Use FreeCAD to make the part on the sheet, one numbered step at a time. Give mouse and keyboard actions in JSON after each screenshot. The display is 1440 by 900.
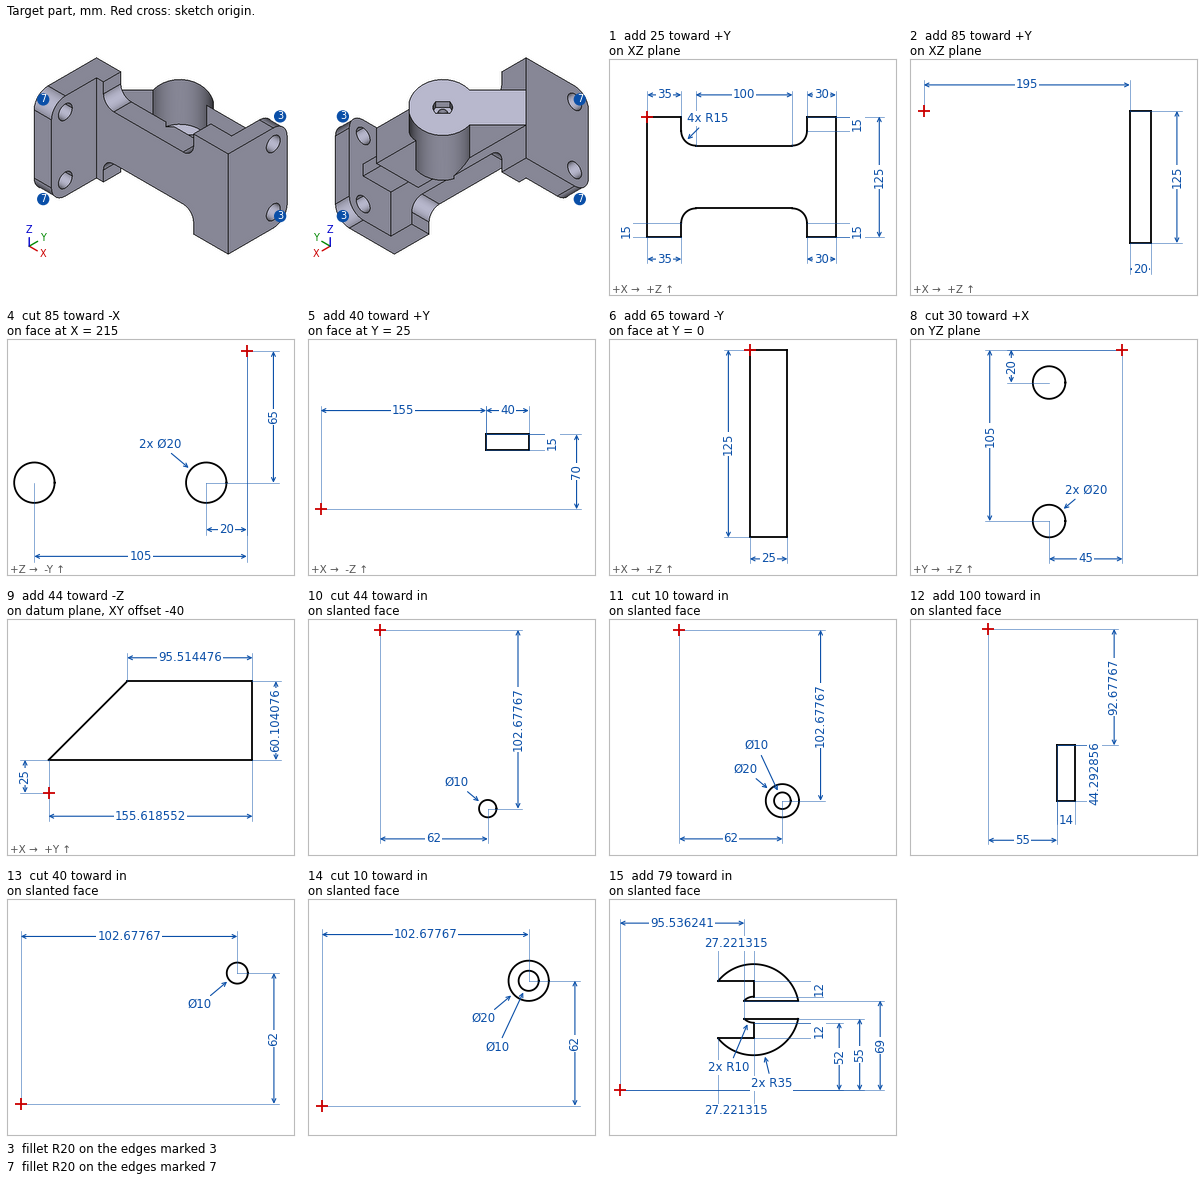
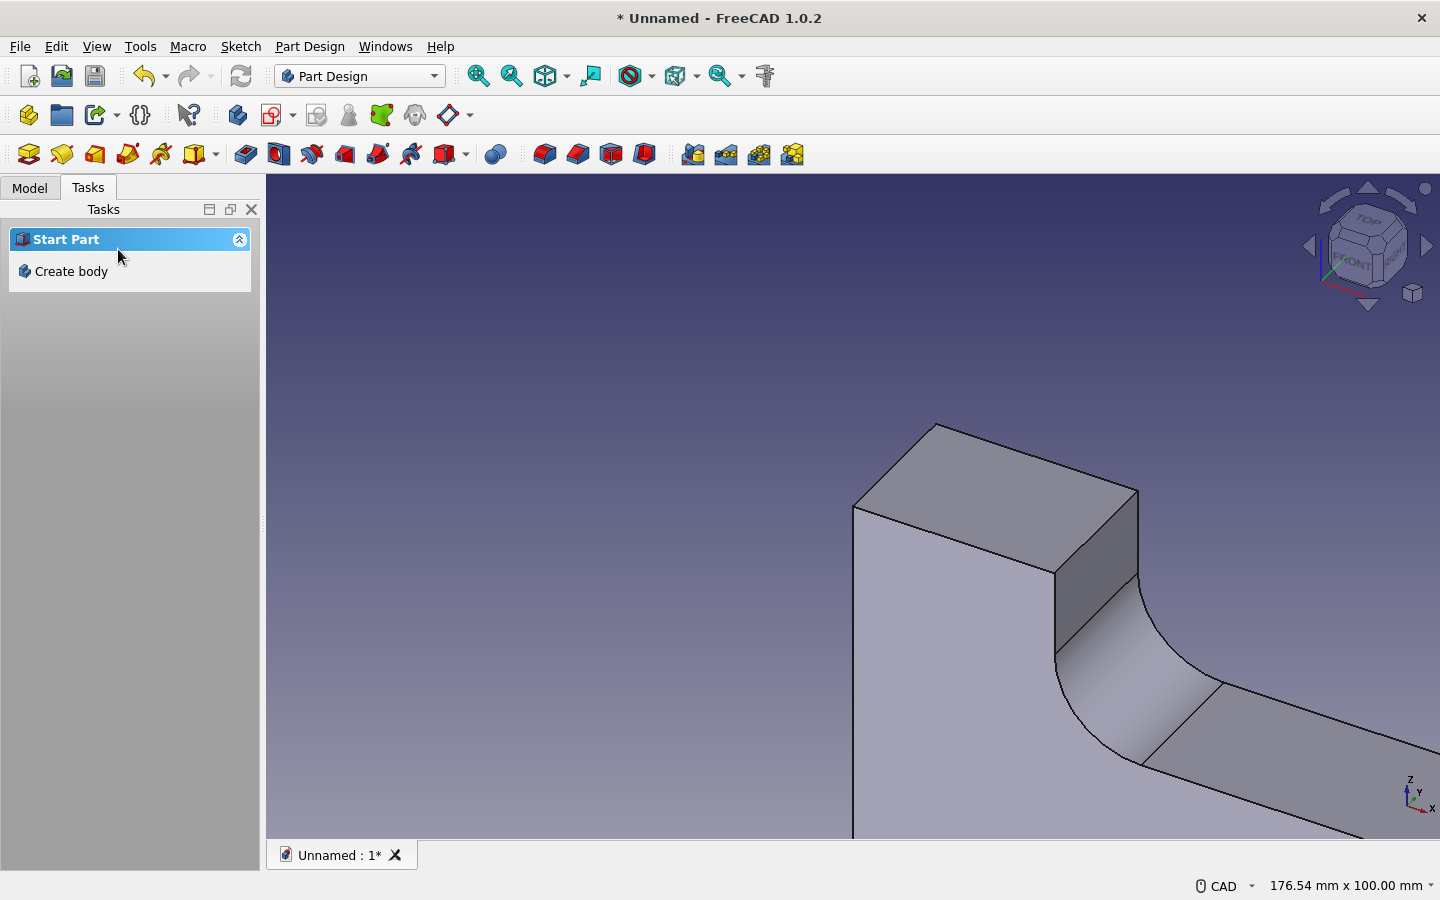
{"action": "left_click", "coordinate": [479, 76]}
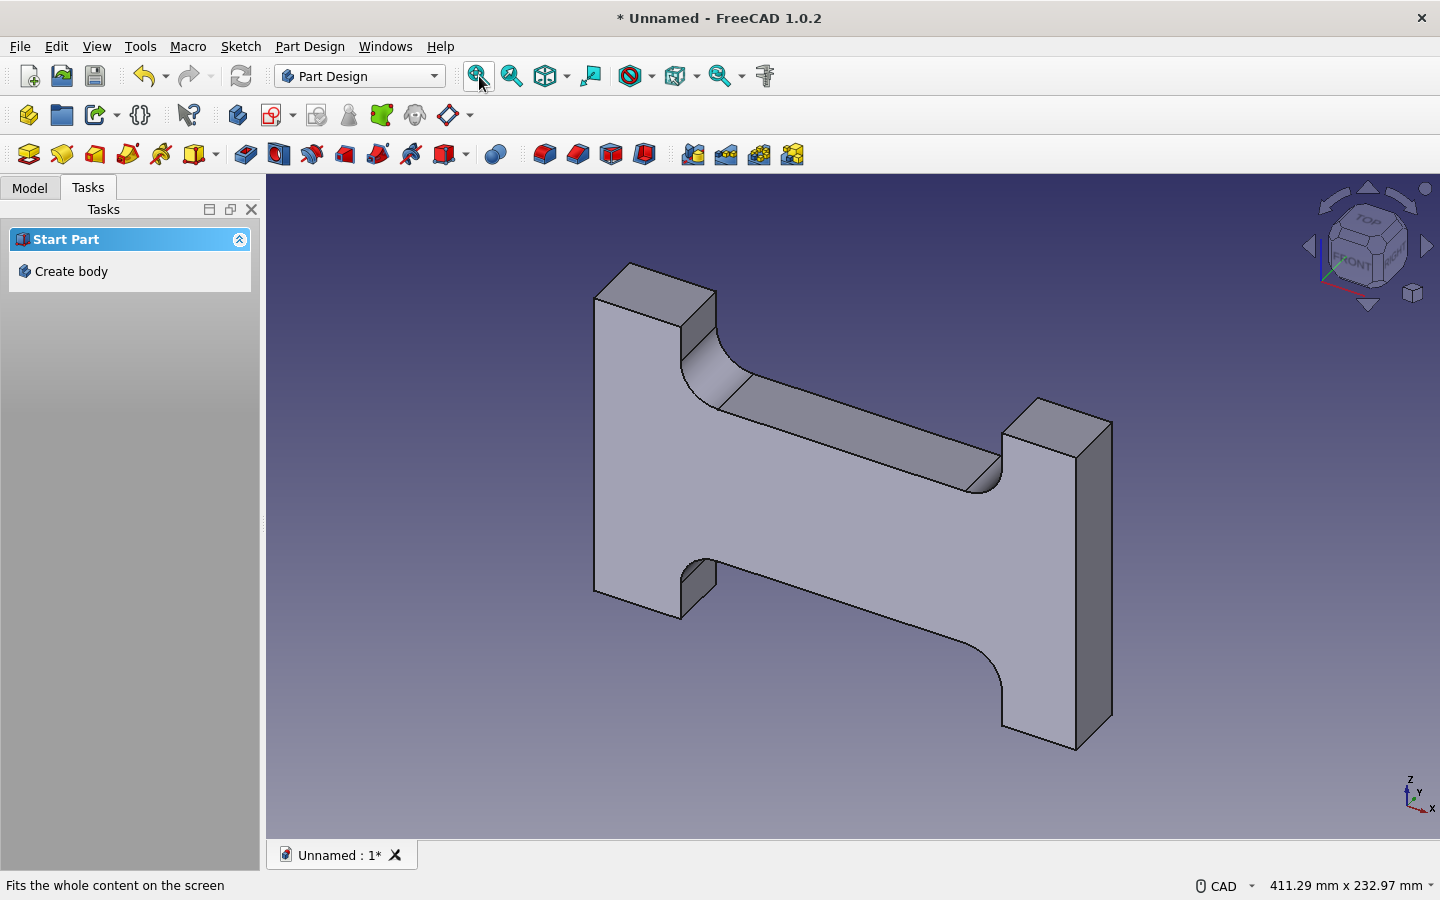
{"action": "left_click", "coordinate": [270, 116]}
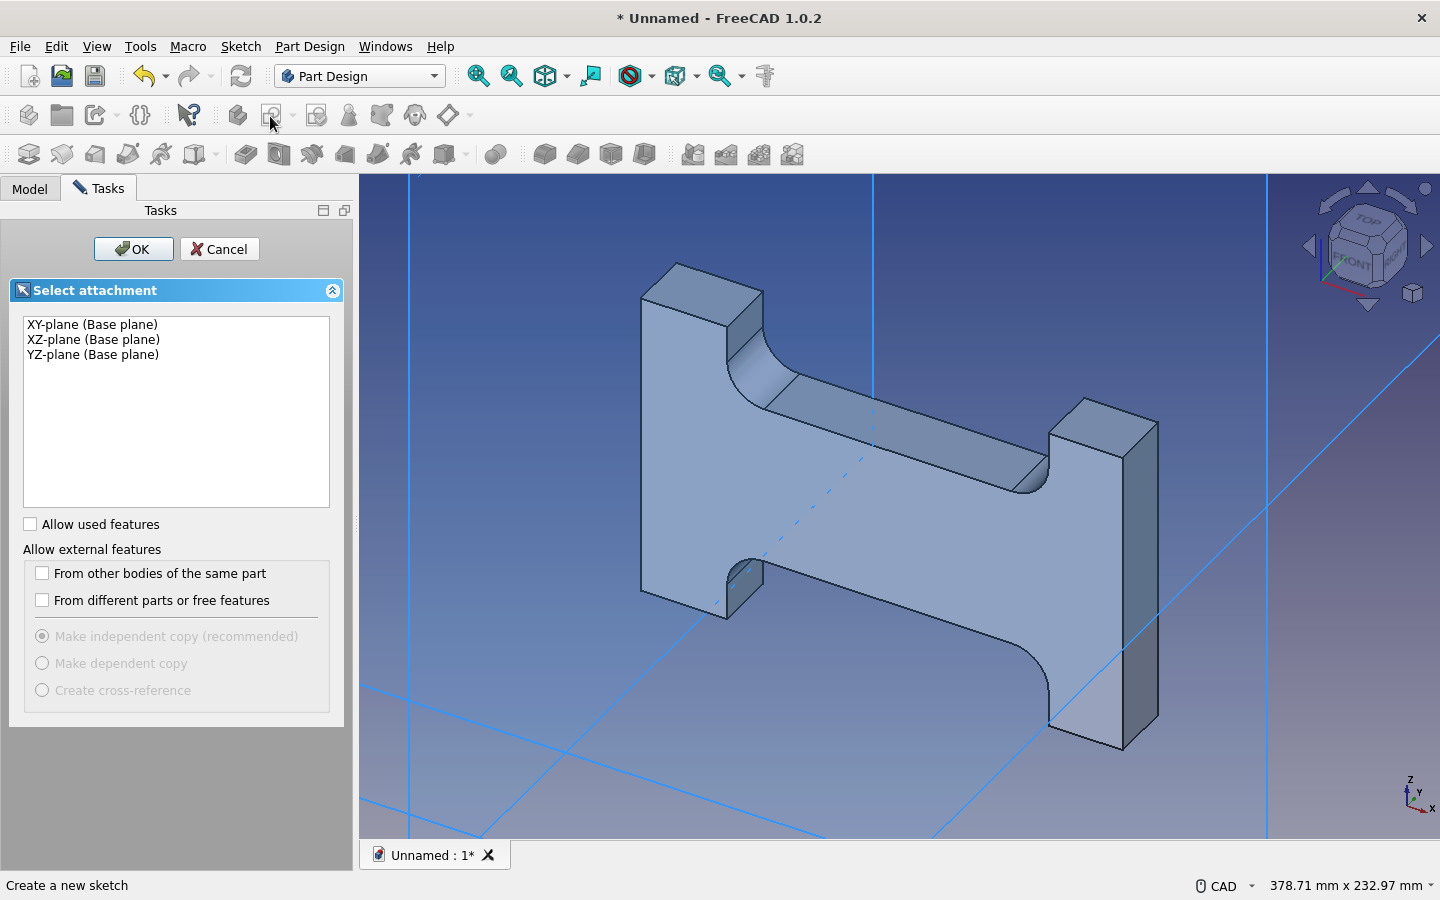
{"action": "left_click", "coordinate": [84, 340]}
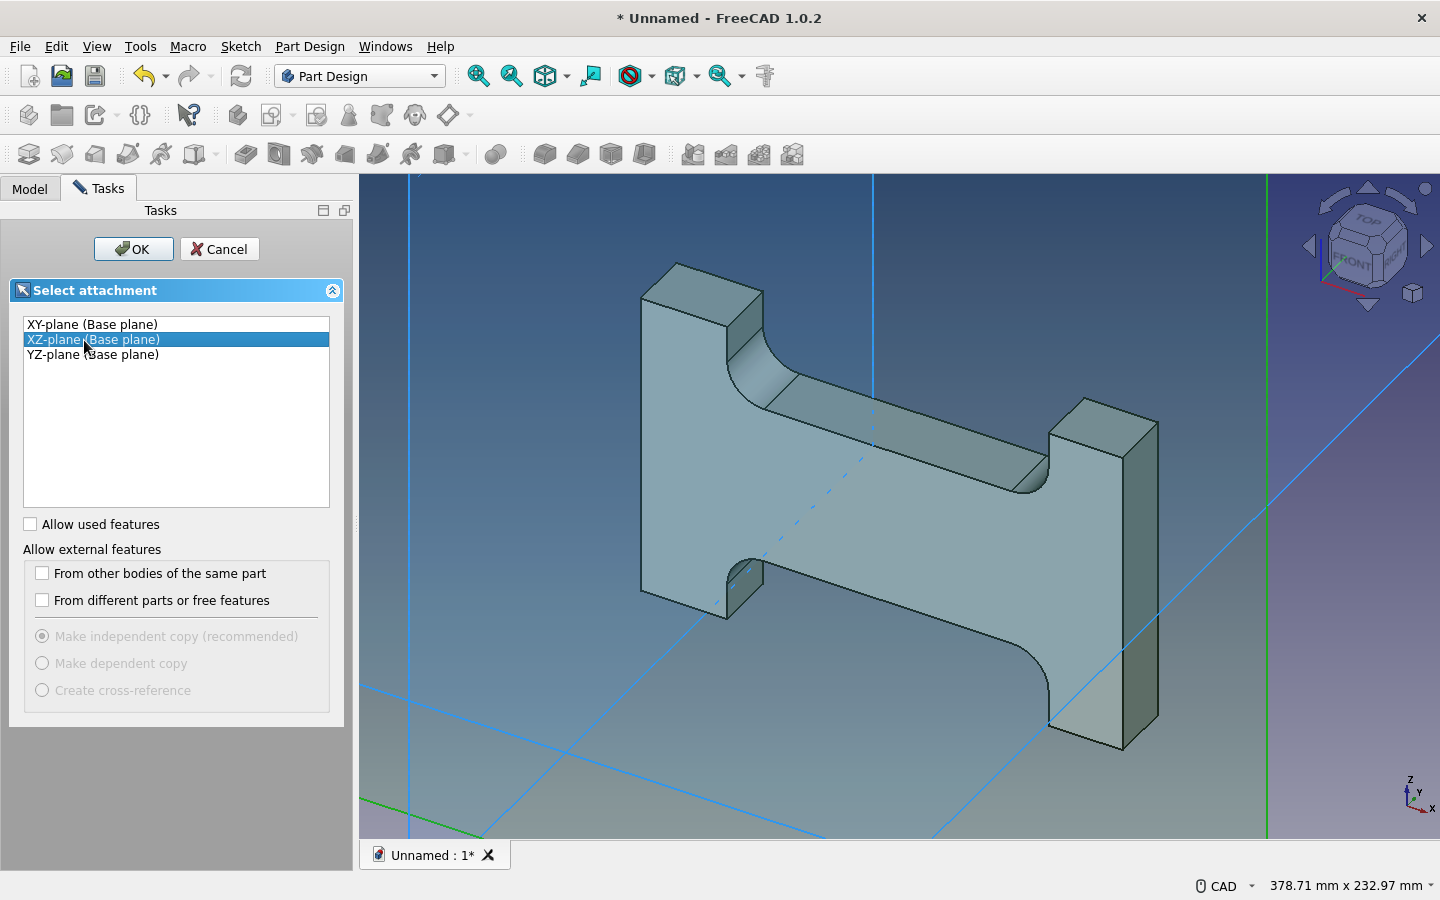
{"action": "left_click", "coordinate": [134, 249]}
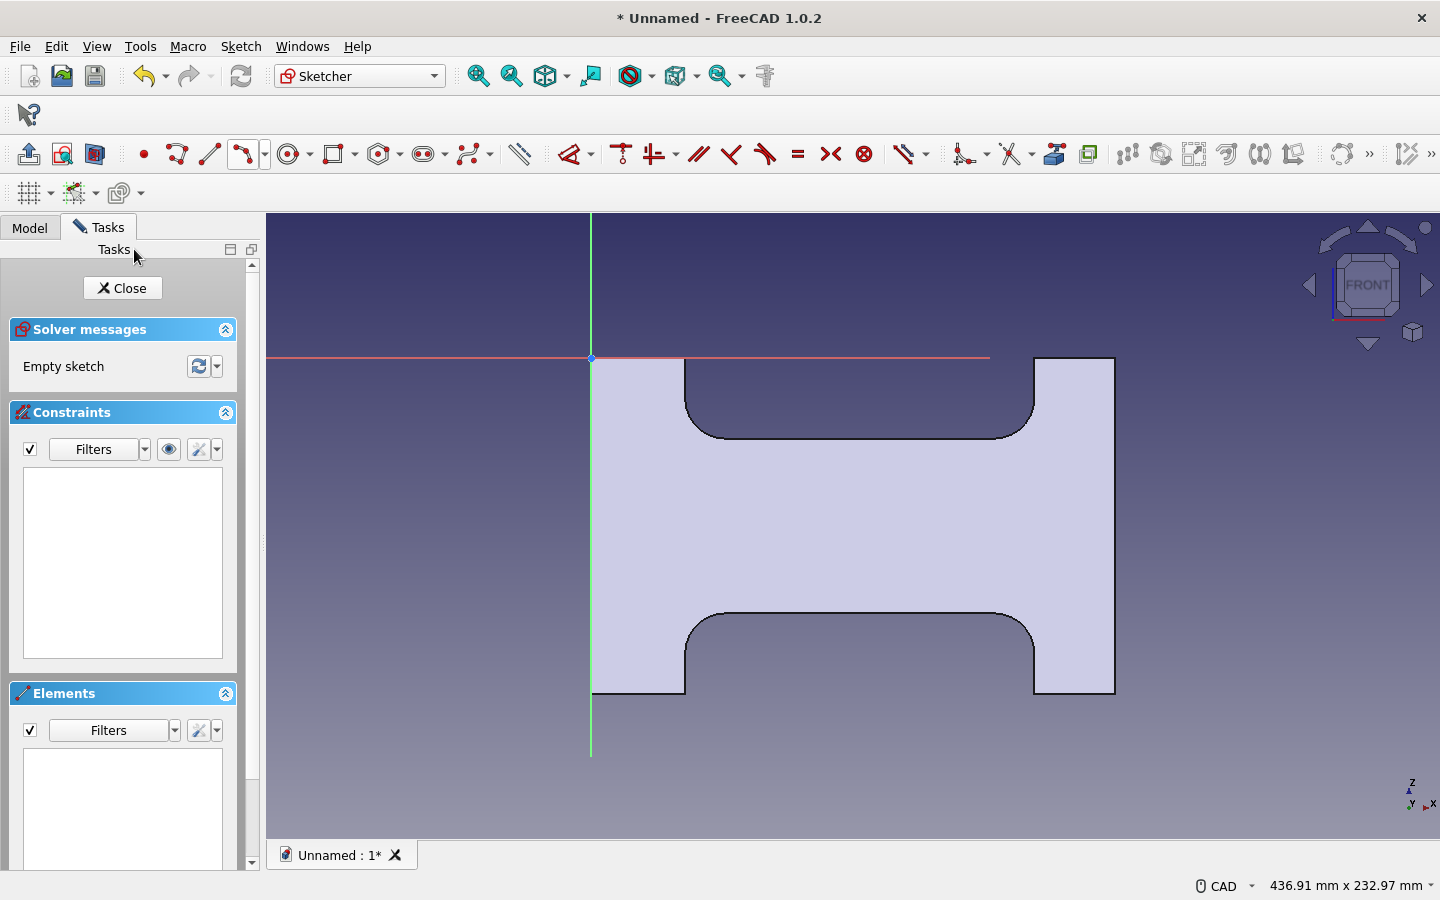
{"action": "left_click", "coordinate": [332, 154]}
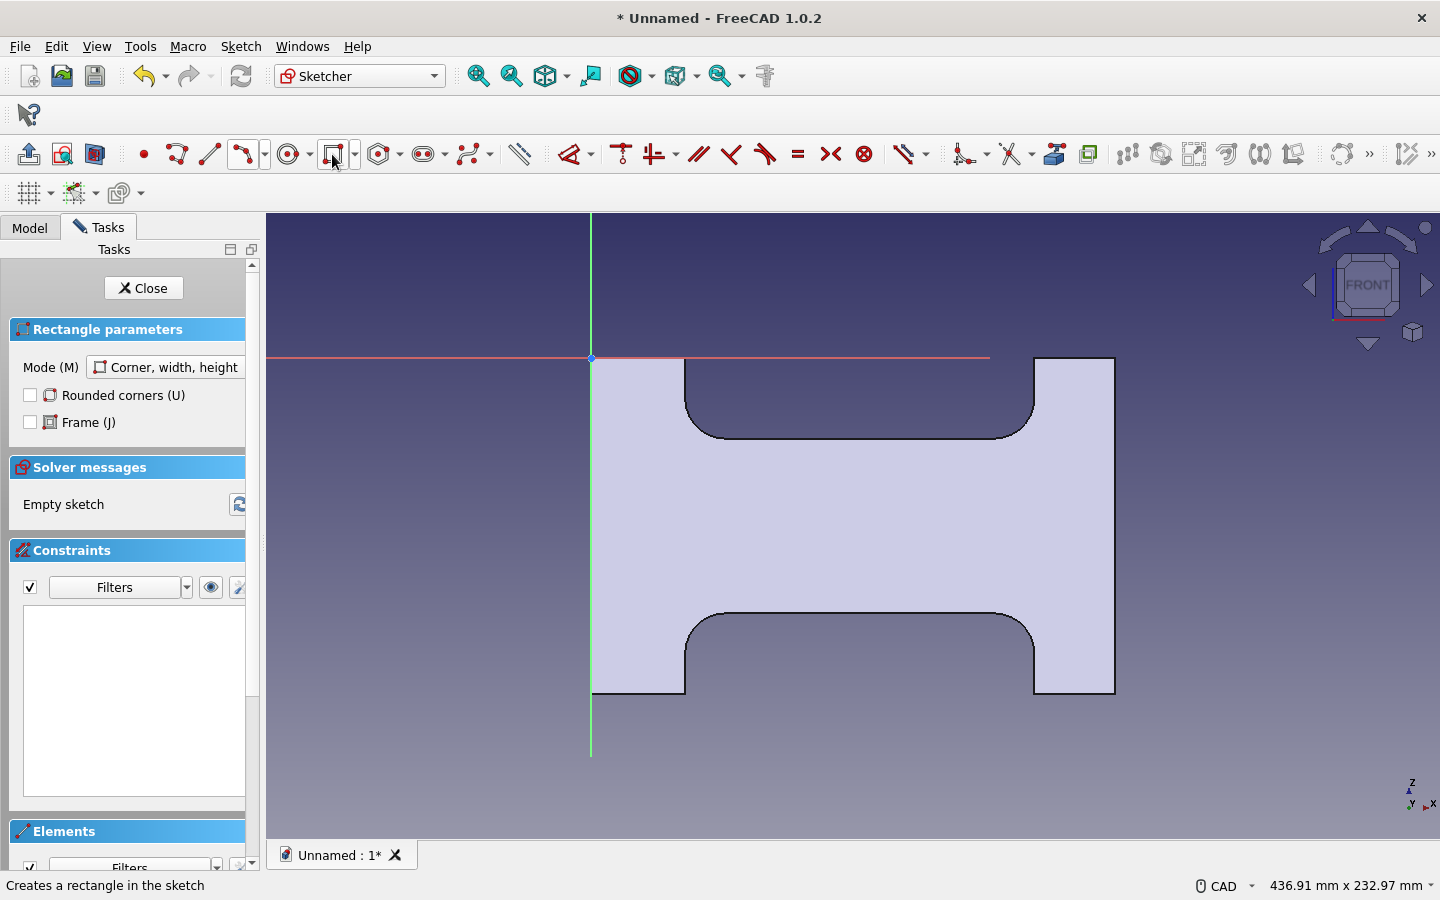
{"action": "left_click", "coordinate": [1115, 358]}
{"action": "left_click", "coordinate": [1169, 694]}
{"action": "key", "text": "Escape"}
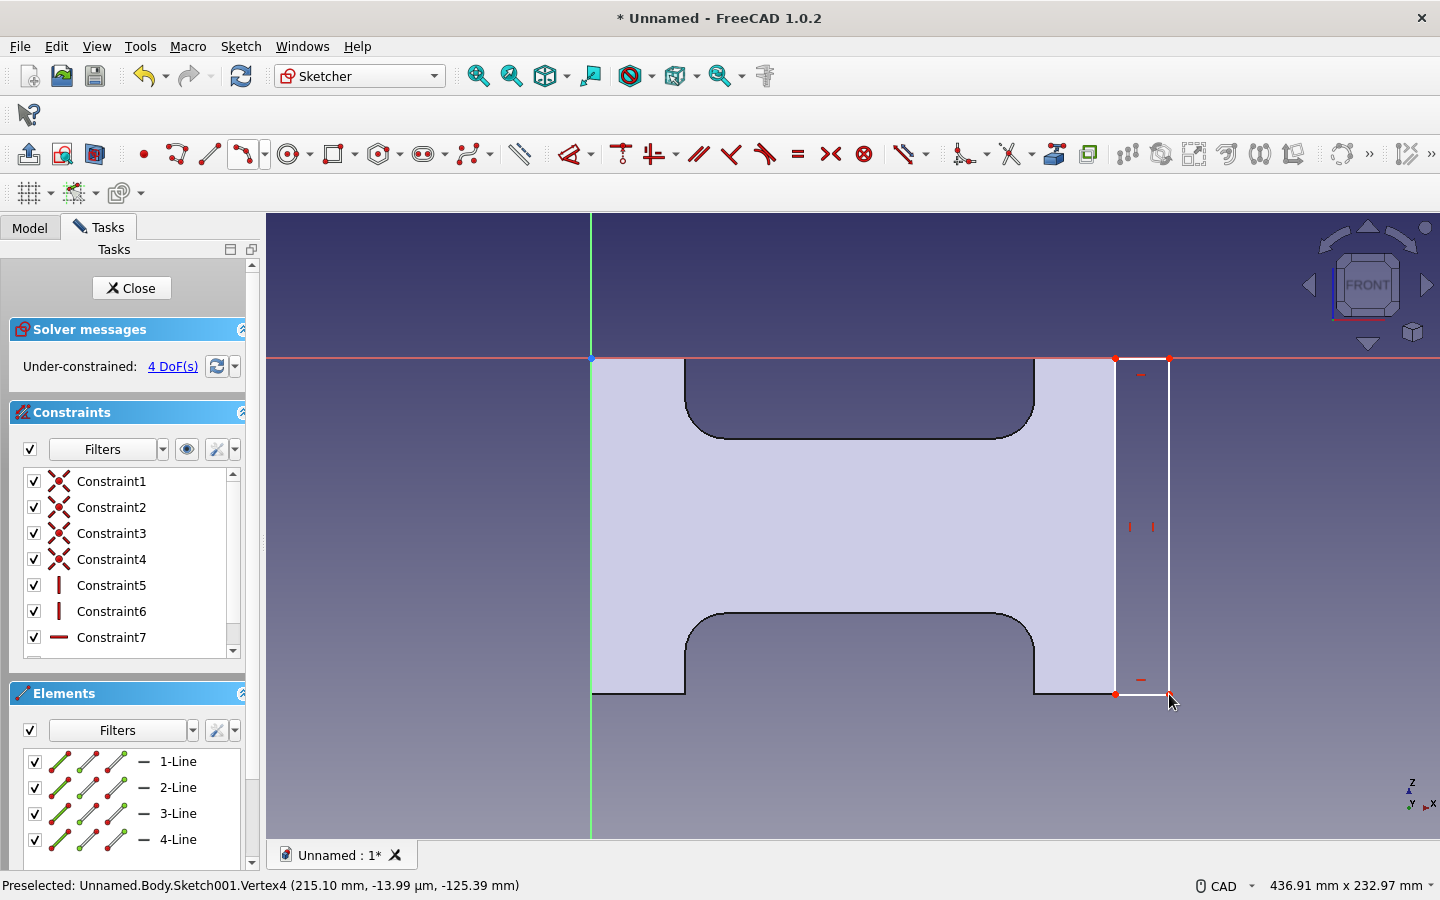
{"action": "left_click", "coordinate": [1115, 359]}